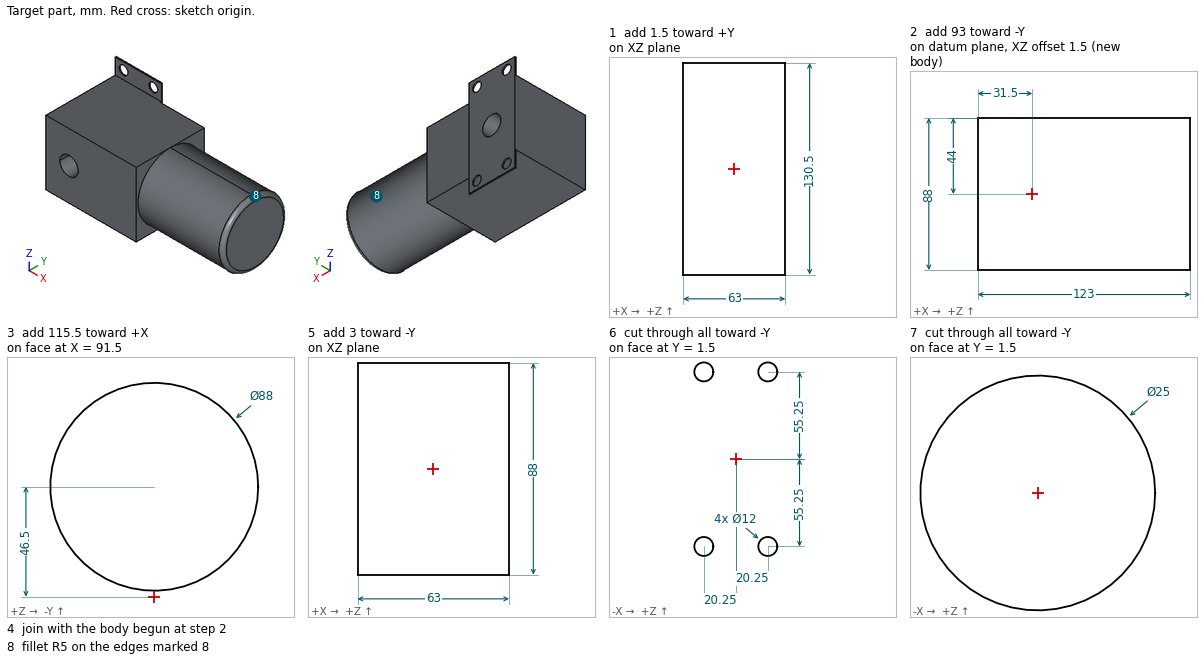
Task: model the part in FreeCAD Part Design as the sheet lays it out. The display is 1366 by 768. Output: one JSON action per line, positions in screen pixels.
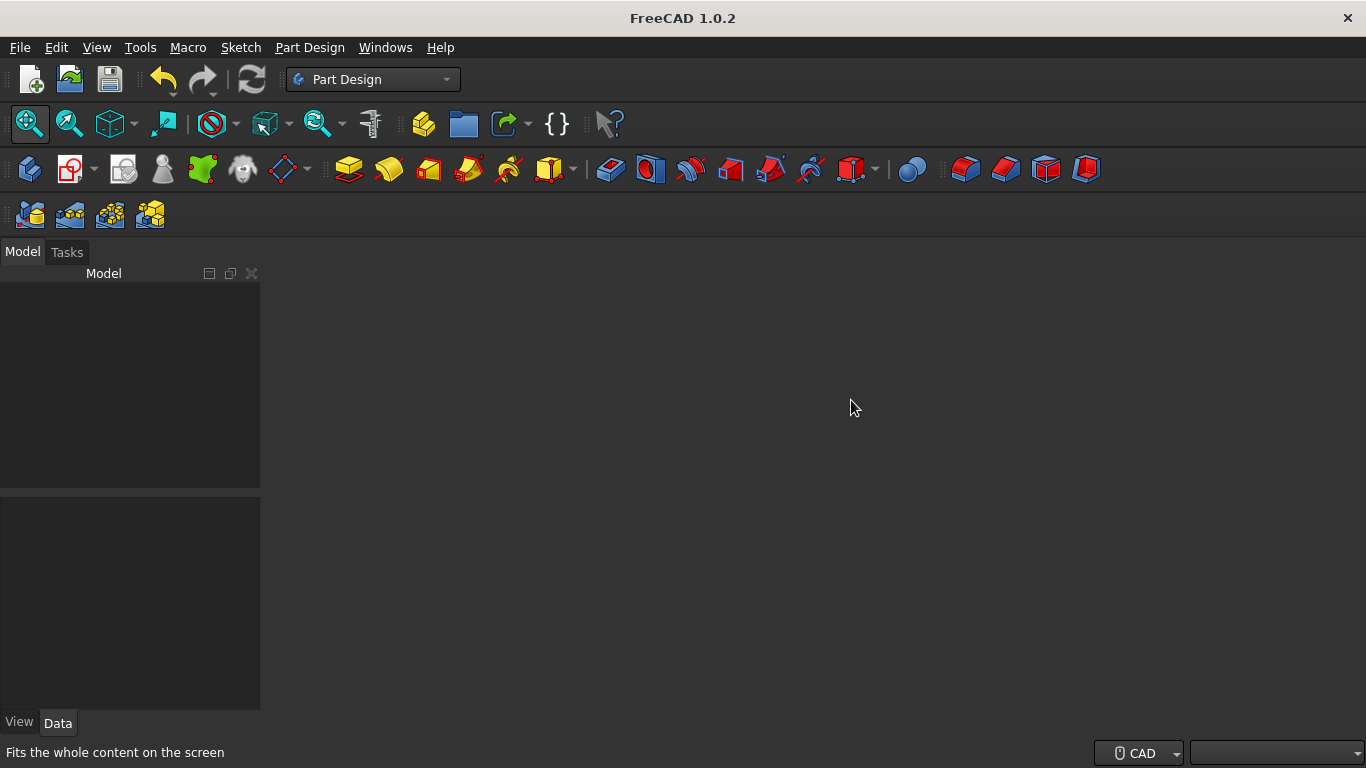
{"action": "left_click", "coordinate": [30, 80]}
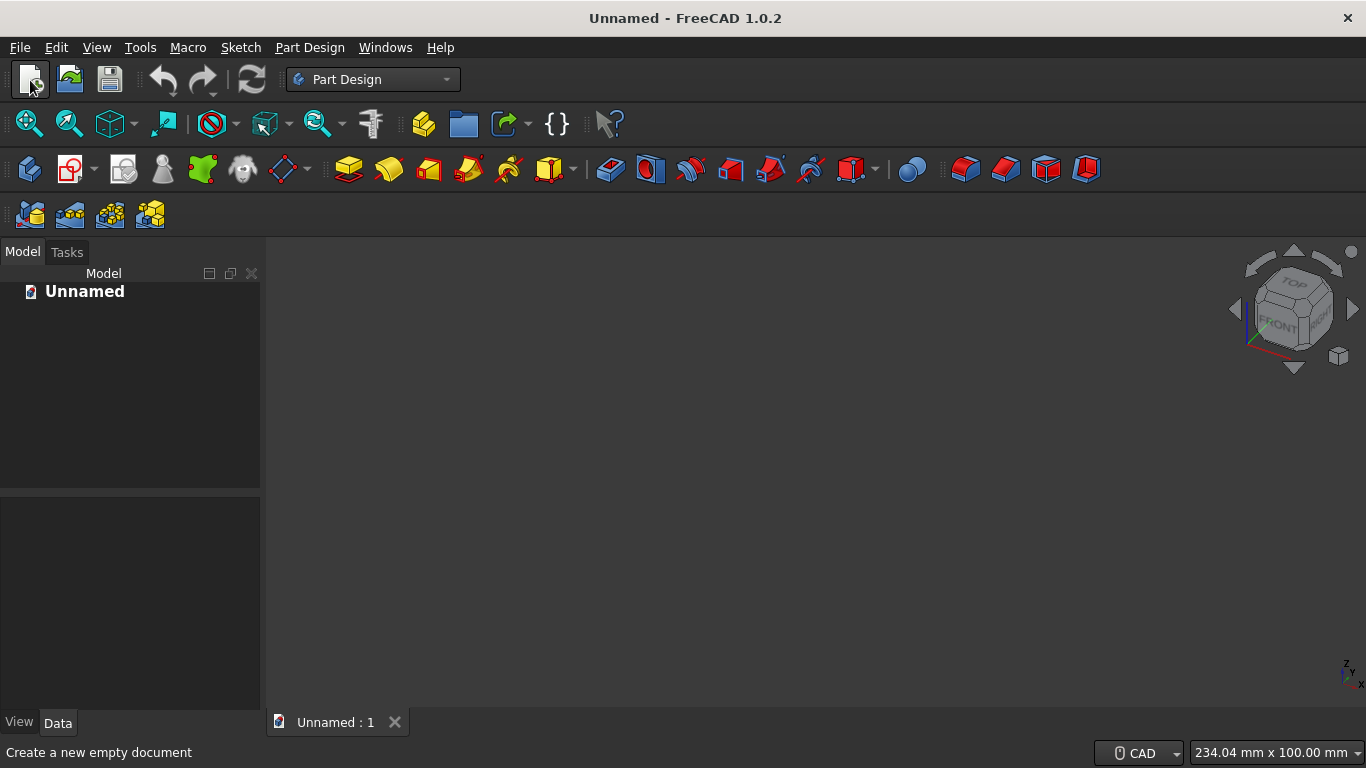
{"action": "left_click", "coordinate": [70, 170]}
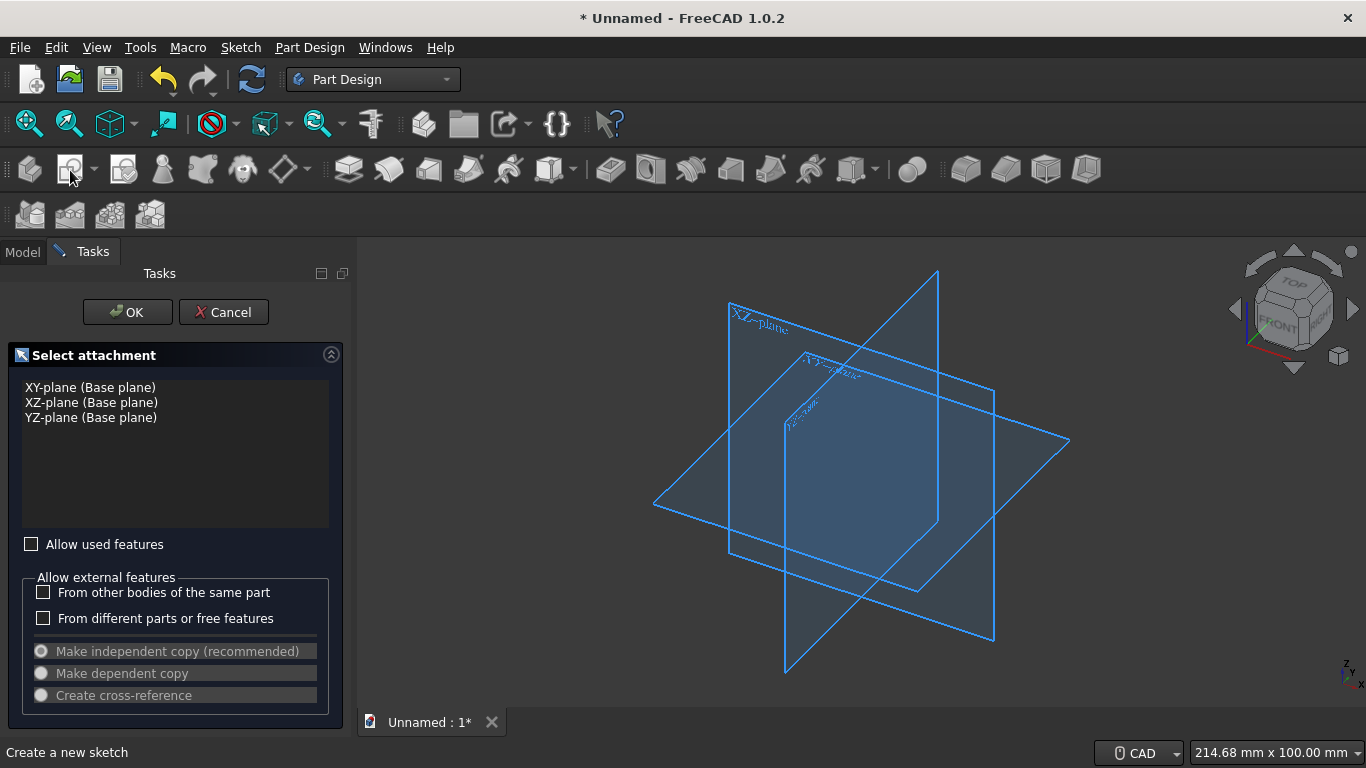
{"action": "left_click", "coordinate": [82, 402]}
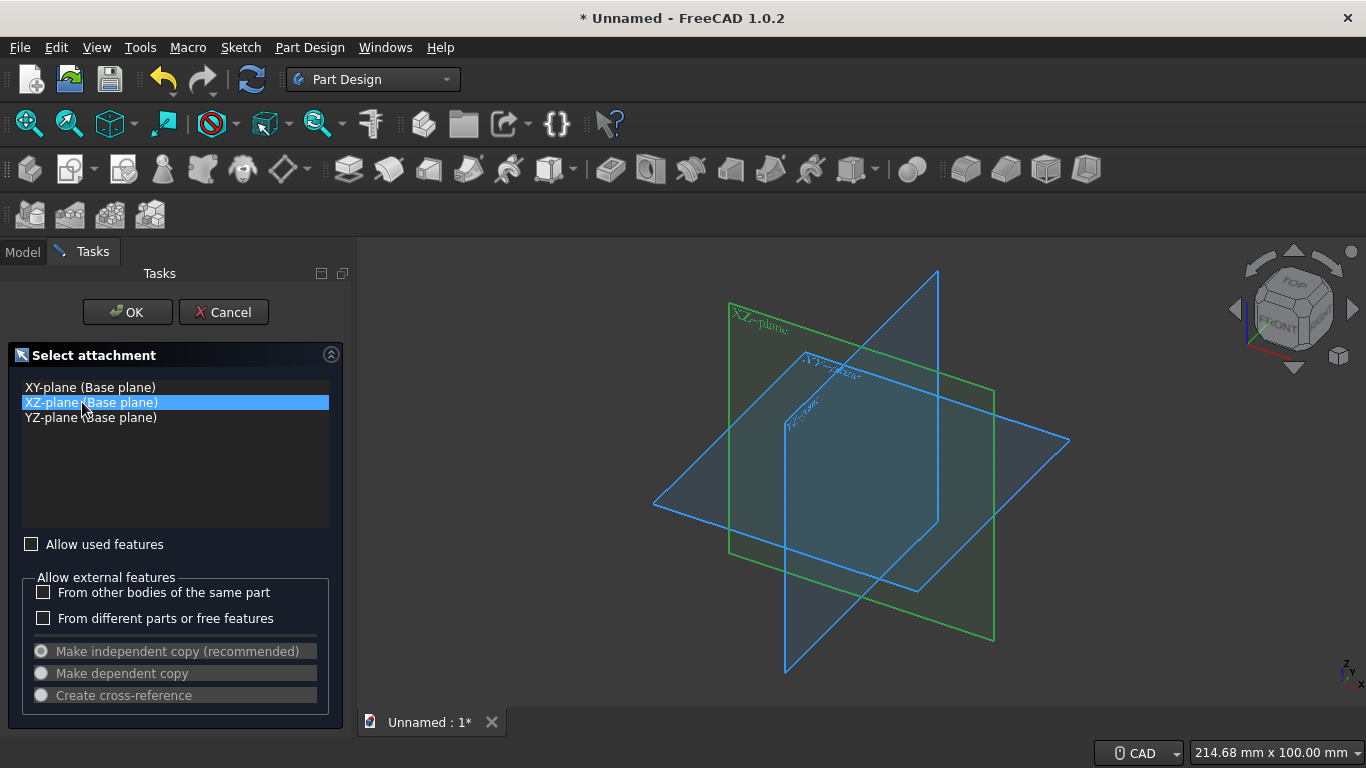
{"action": "left_click", "coordinate": [128, 312]}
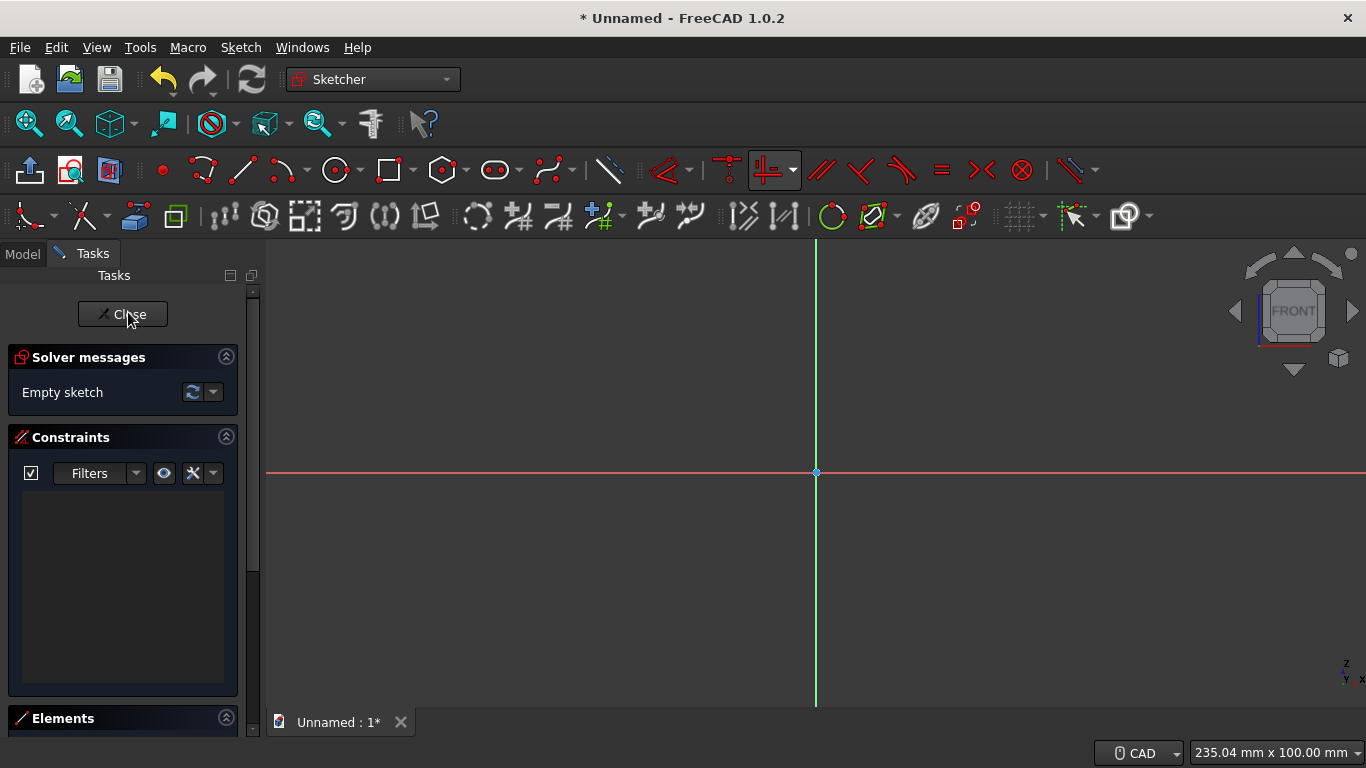
{"action": "scroll", "coordinate": [692, 473], "scroll_direction": "down", "scroll_amount": 4}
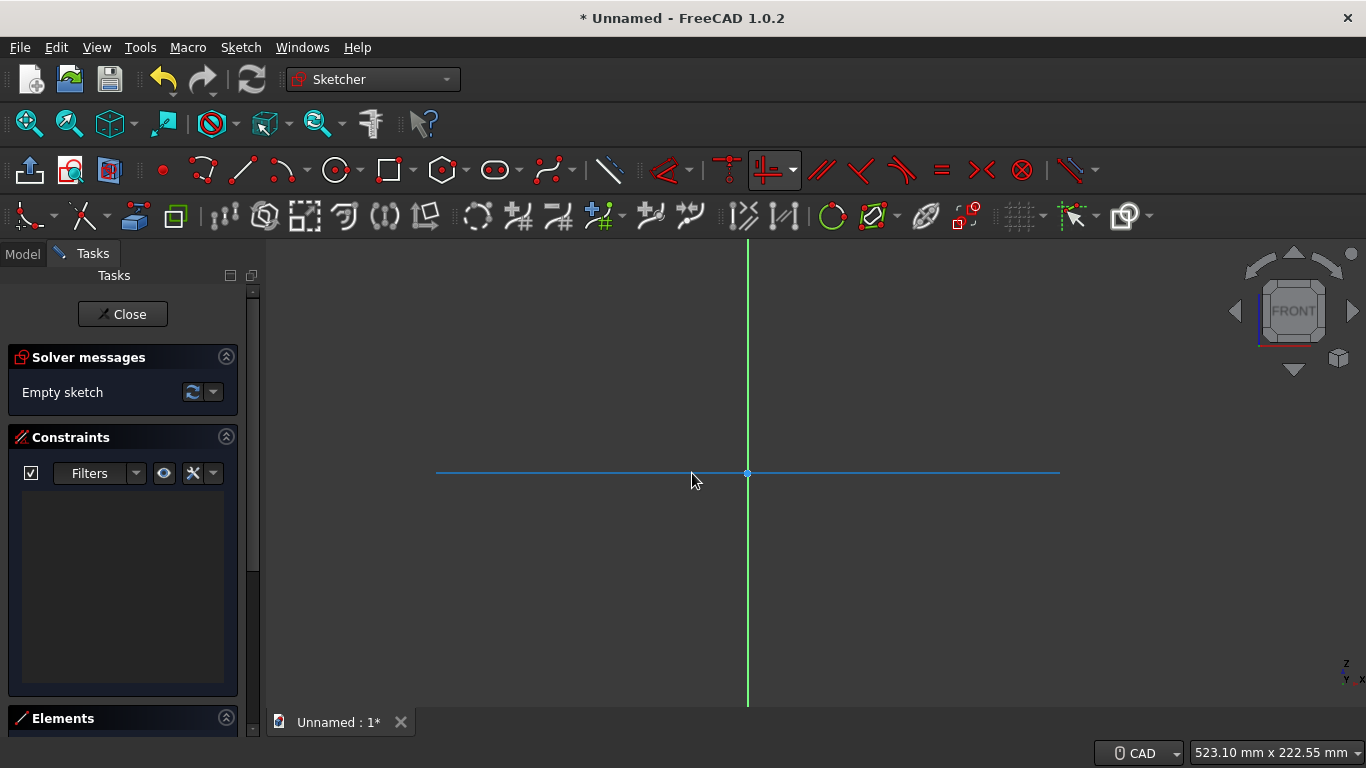
{"action": "key", "text": "g v"}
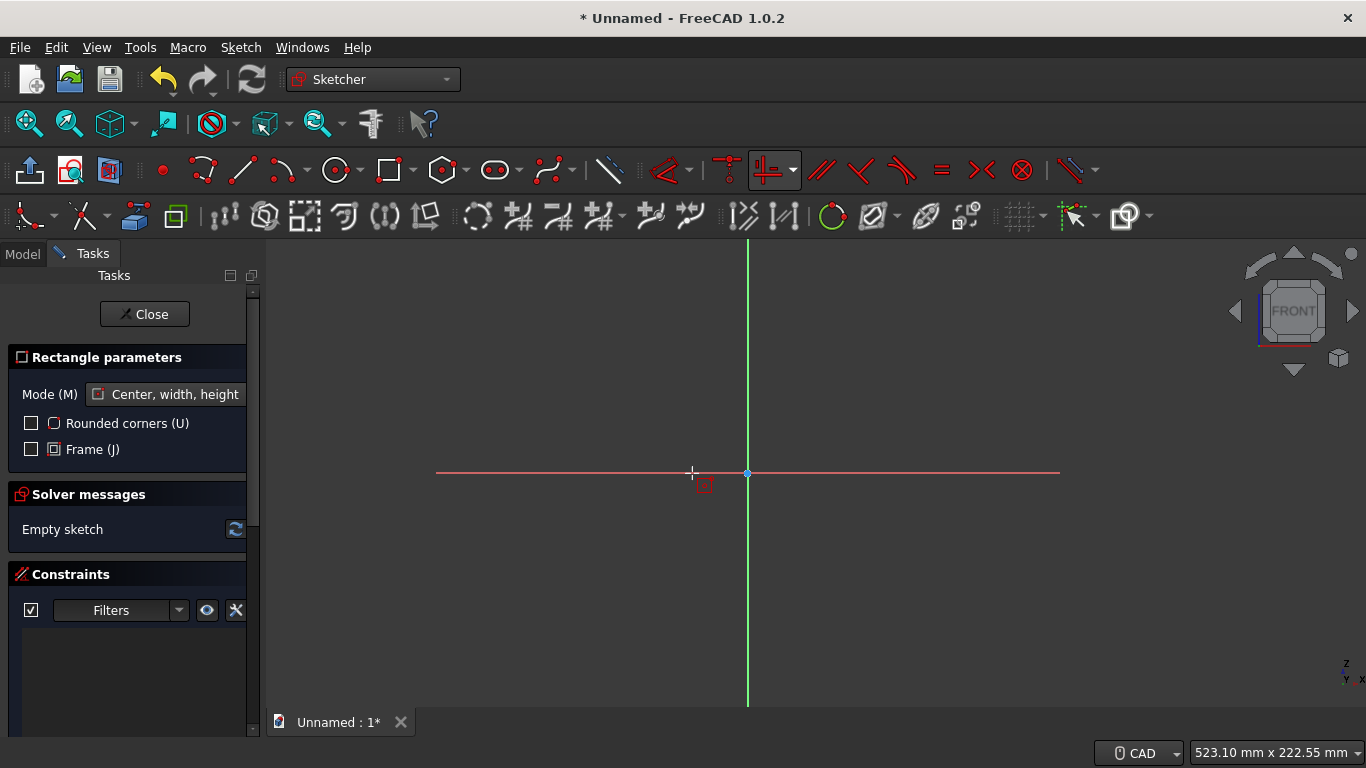
{"action": "left_click", "coordinate": [748, 473]}
{"action": "left_click", "coordinate": [814, 336]}
{"action": "key", "text": "Escape"}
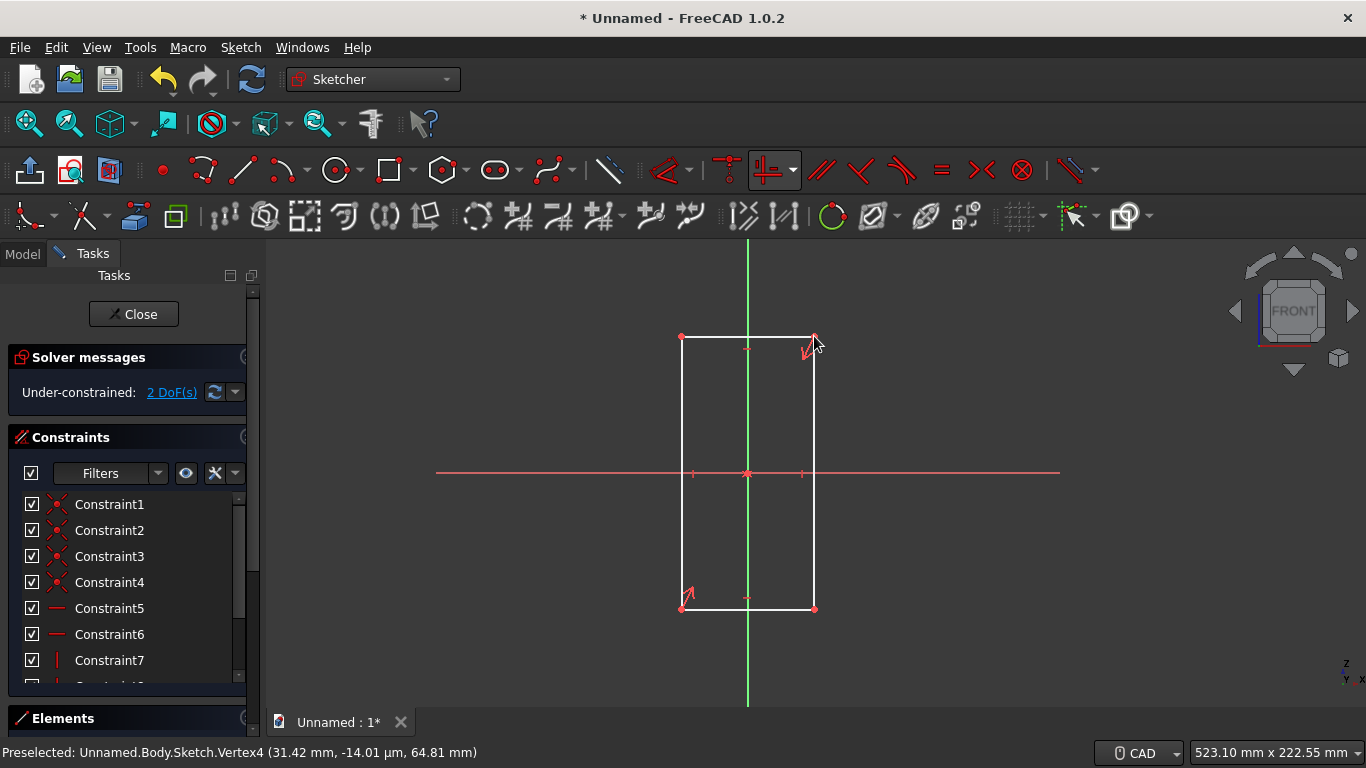
{"action": "left_click", "coordinate": [664, 170]}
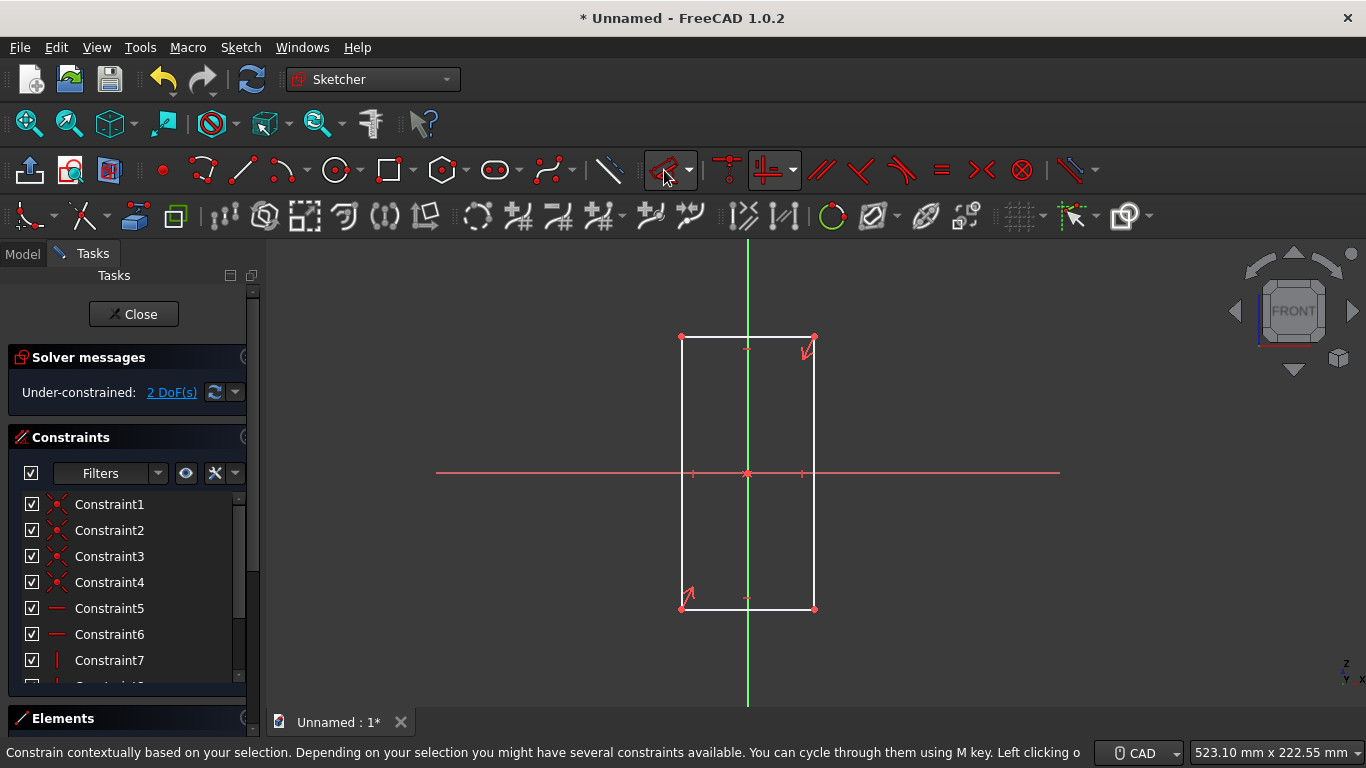
{"action": "left_click", "coordinate": [722, 610]}
{"action": "left_click", "coordinate": [718, 644]}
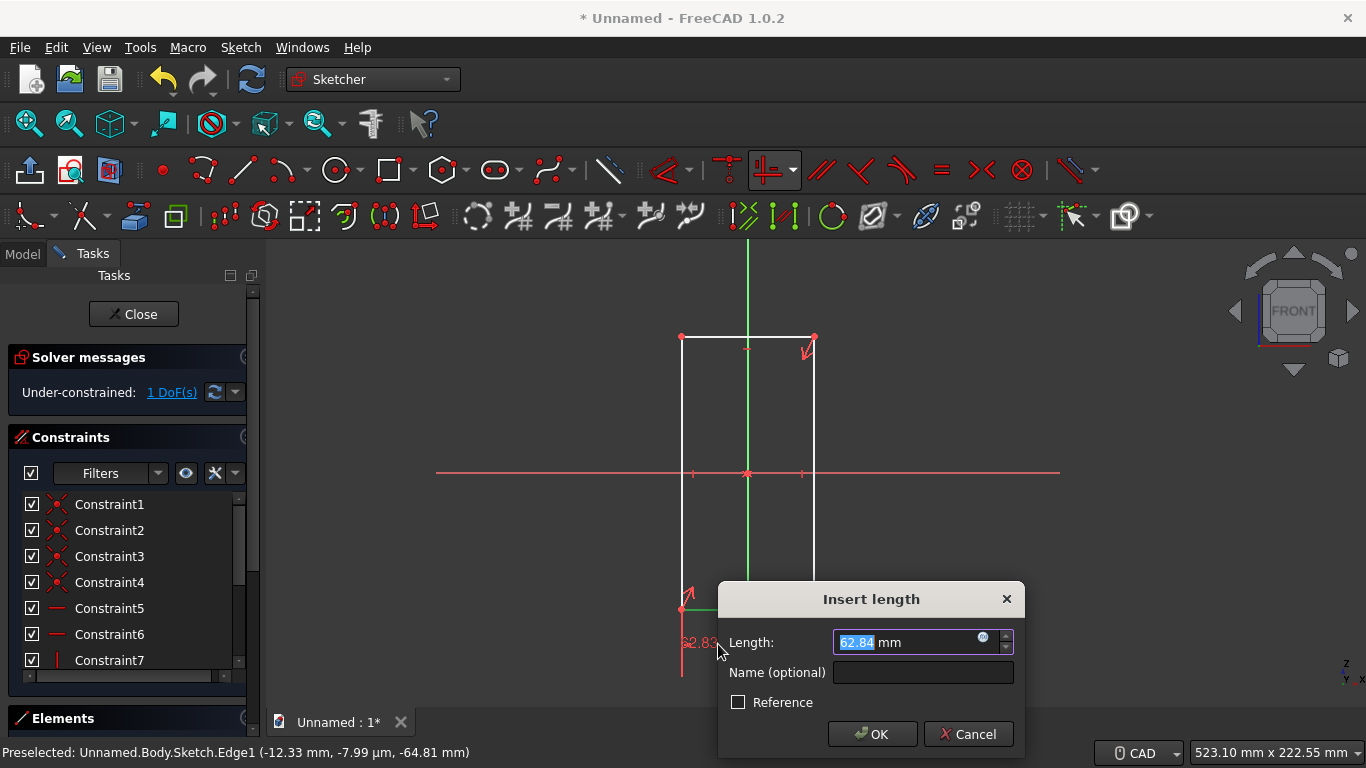
{"action": "type", "text": "63"}
{"action": "key", "text": "Return"}